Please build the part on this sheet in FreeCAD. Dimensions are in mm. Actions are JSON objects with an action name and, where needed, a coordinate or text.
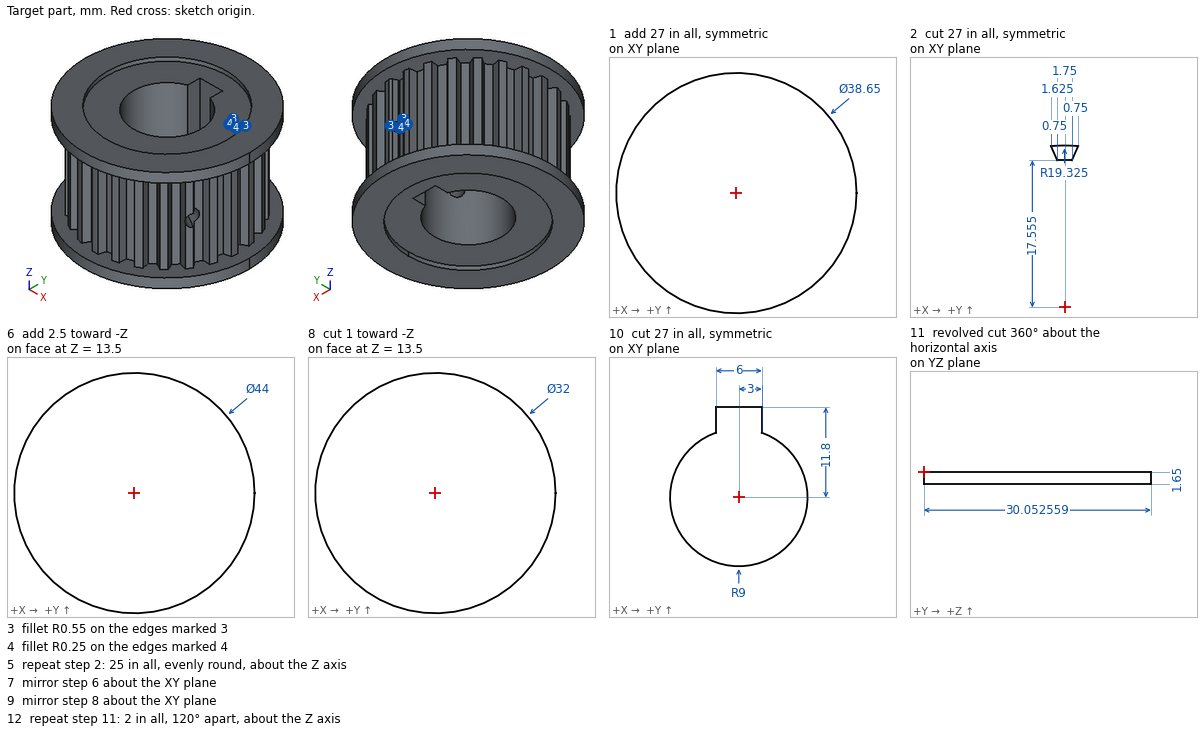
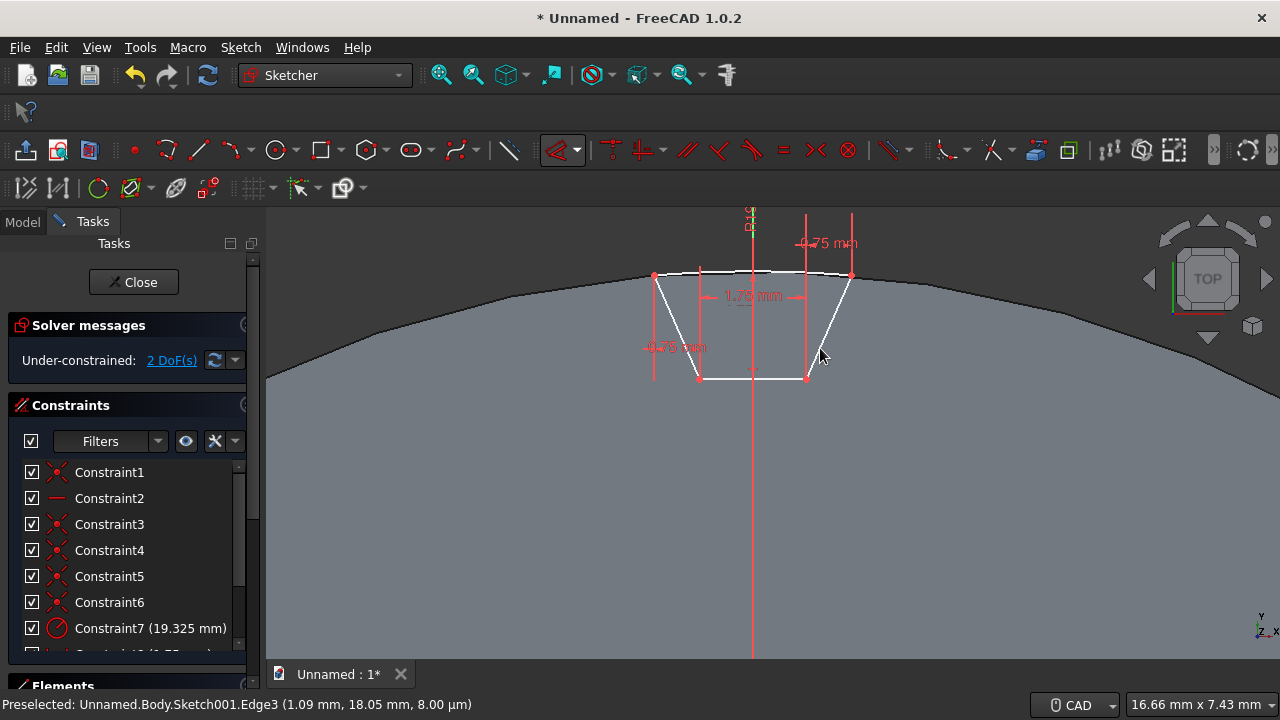
{"action": "left_click", "coordinate": [654, 276]}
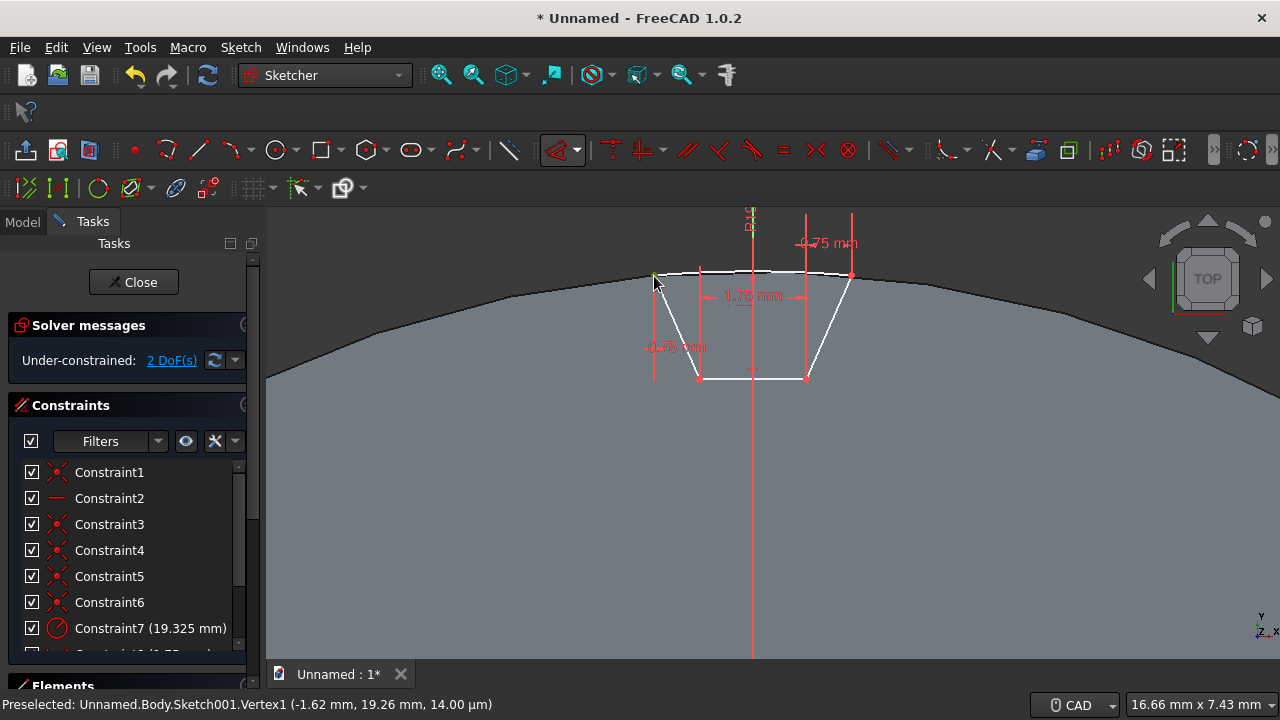
{"action": "left_click", "coordinate": [580, 150]}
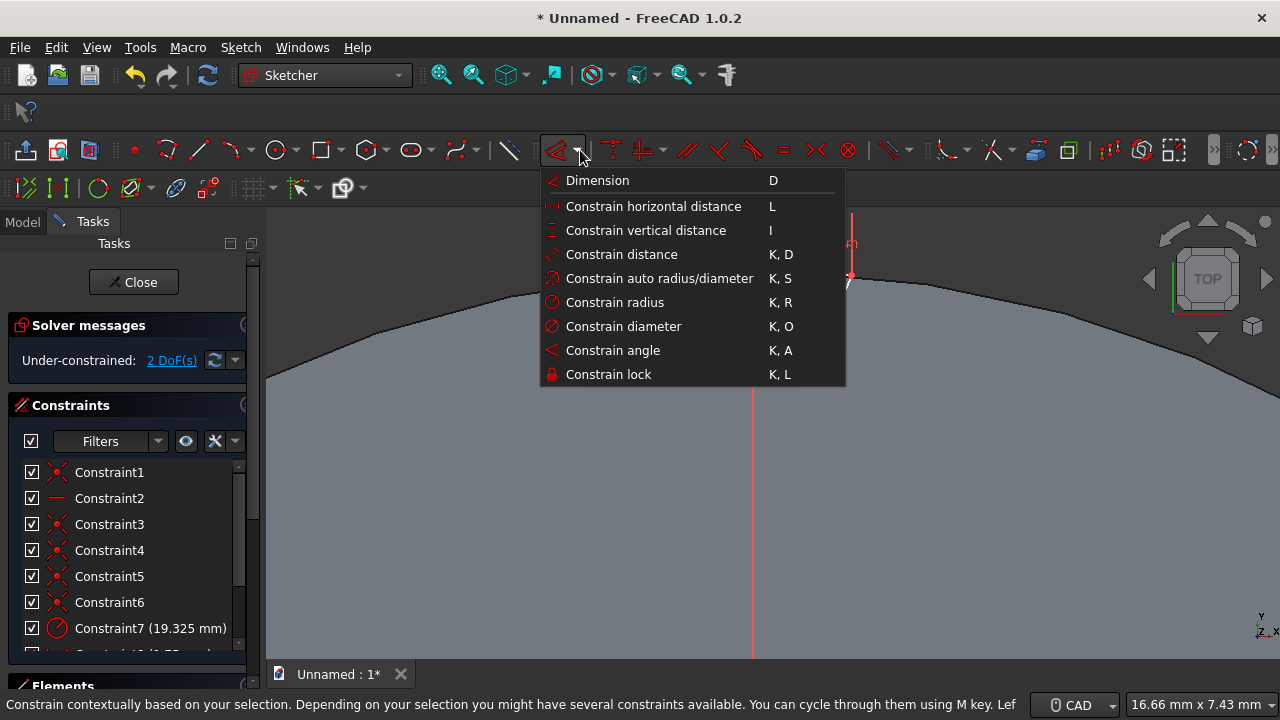
{"action": "left_click", "coordinate": [693, 206]}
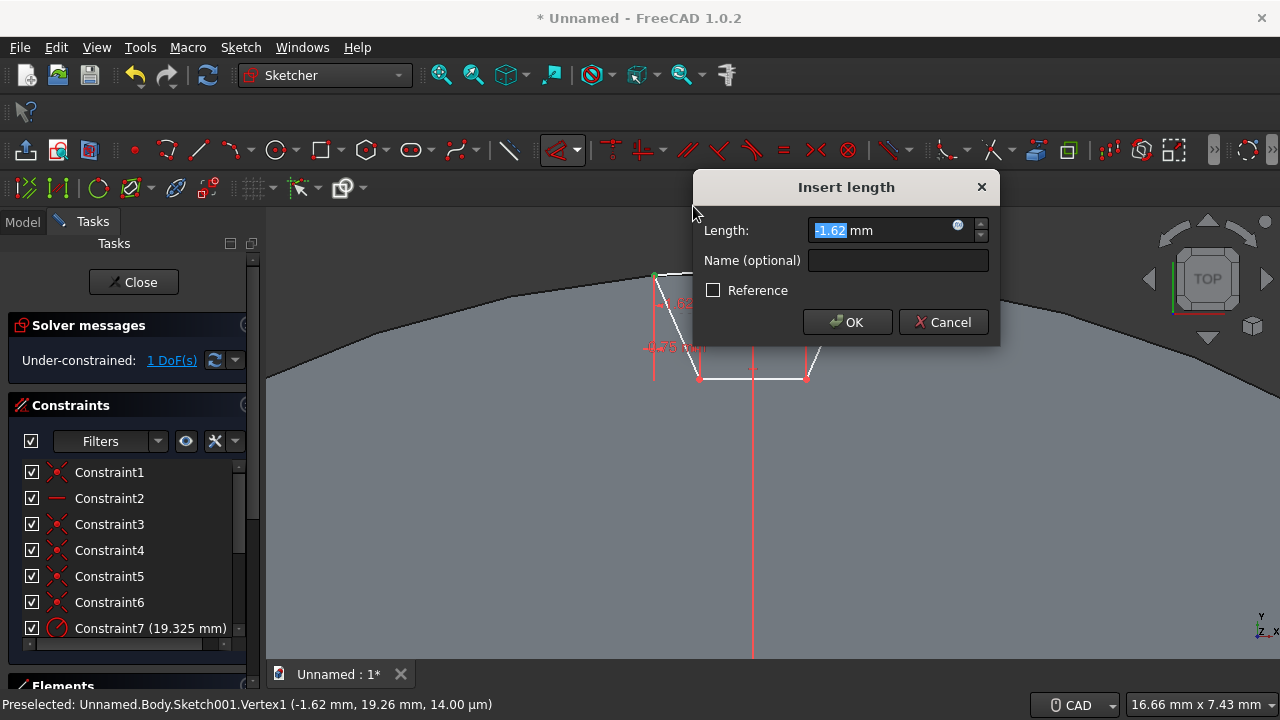
{"action": "type", "text": "-1.625"}
{"action": "key", "text": "Return"}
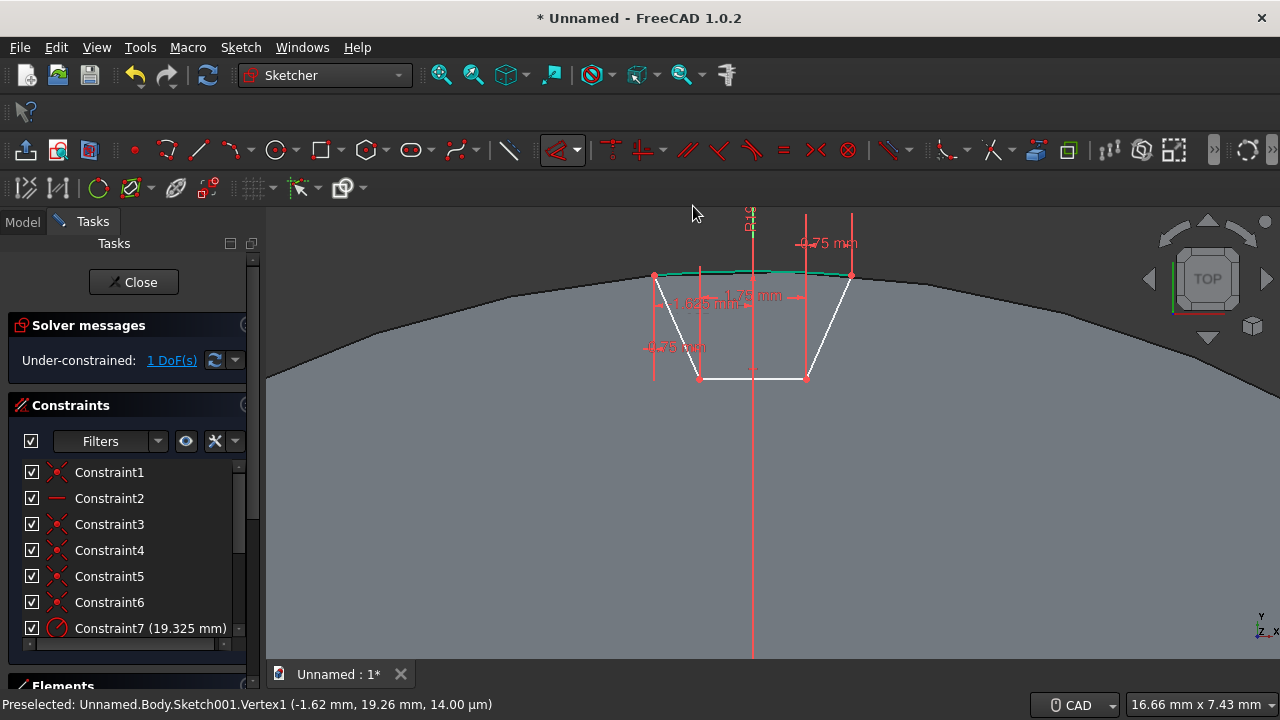
{"action": "left_click", "coordinate": [700, 379]}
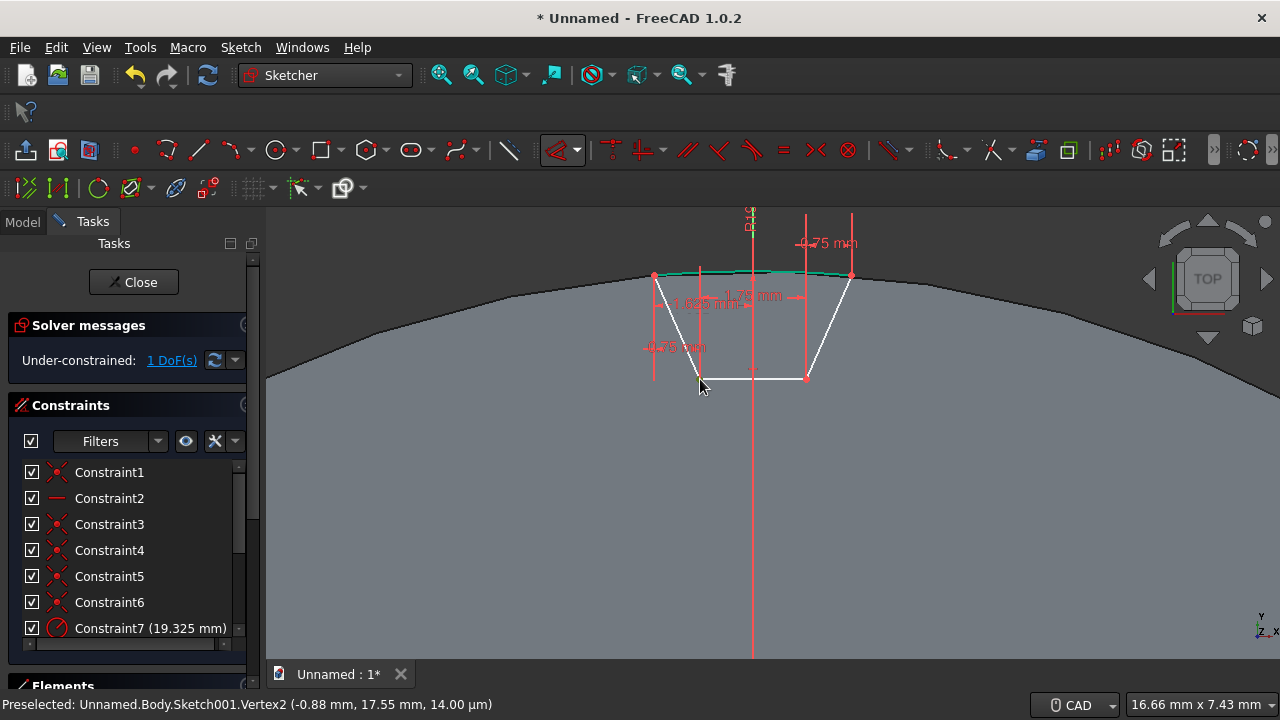
{"action": "left_click", "coordinate": [580, 150]}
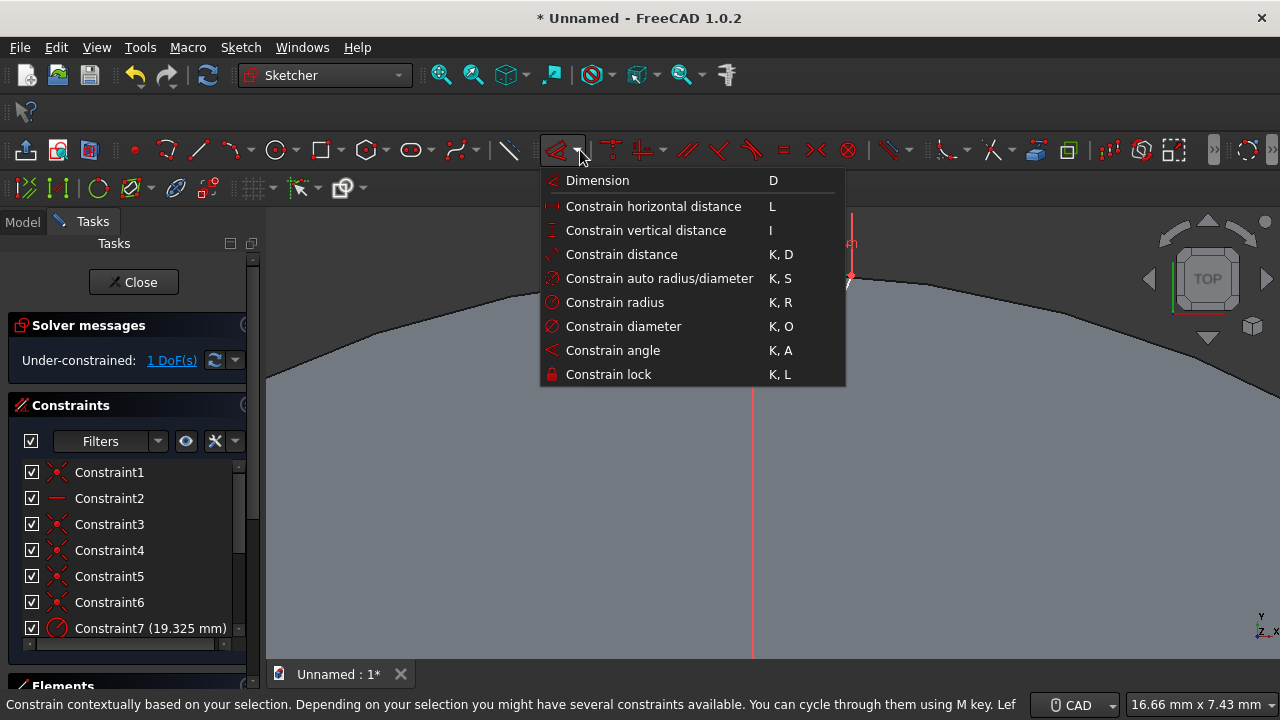
{"action": "left_click", "coordinate": [693, 230]}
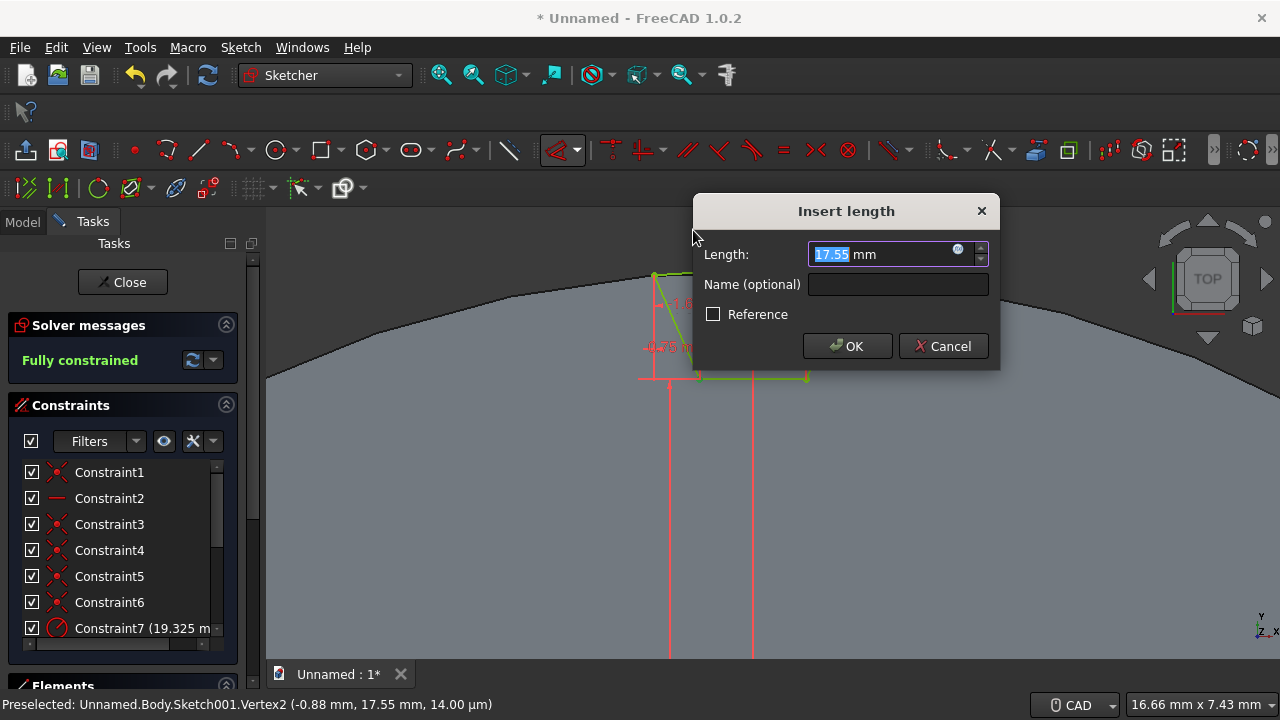
{"action": "type", "text": "17.555"}
{"action": "key", "text": "Return"}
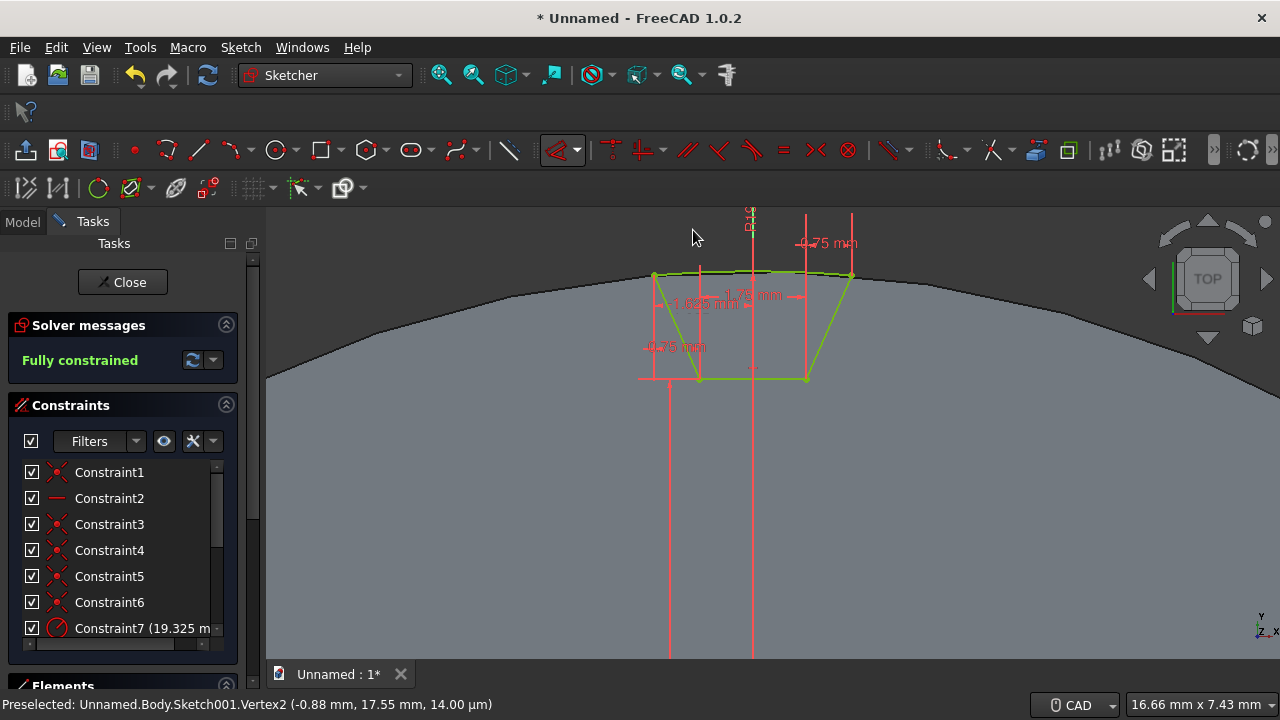
{"action": "left_click", "coordinate": [123, 282]}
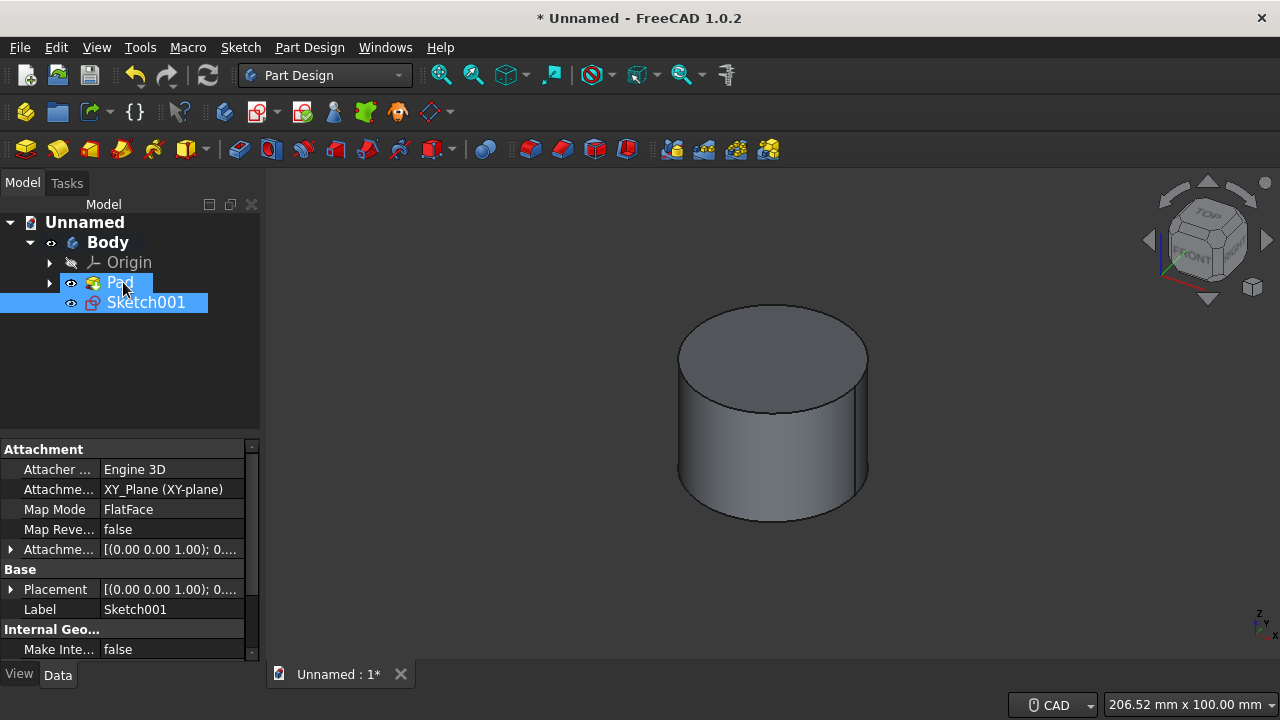
{"action": "left_click", "coordinate": [240, 150]}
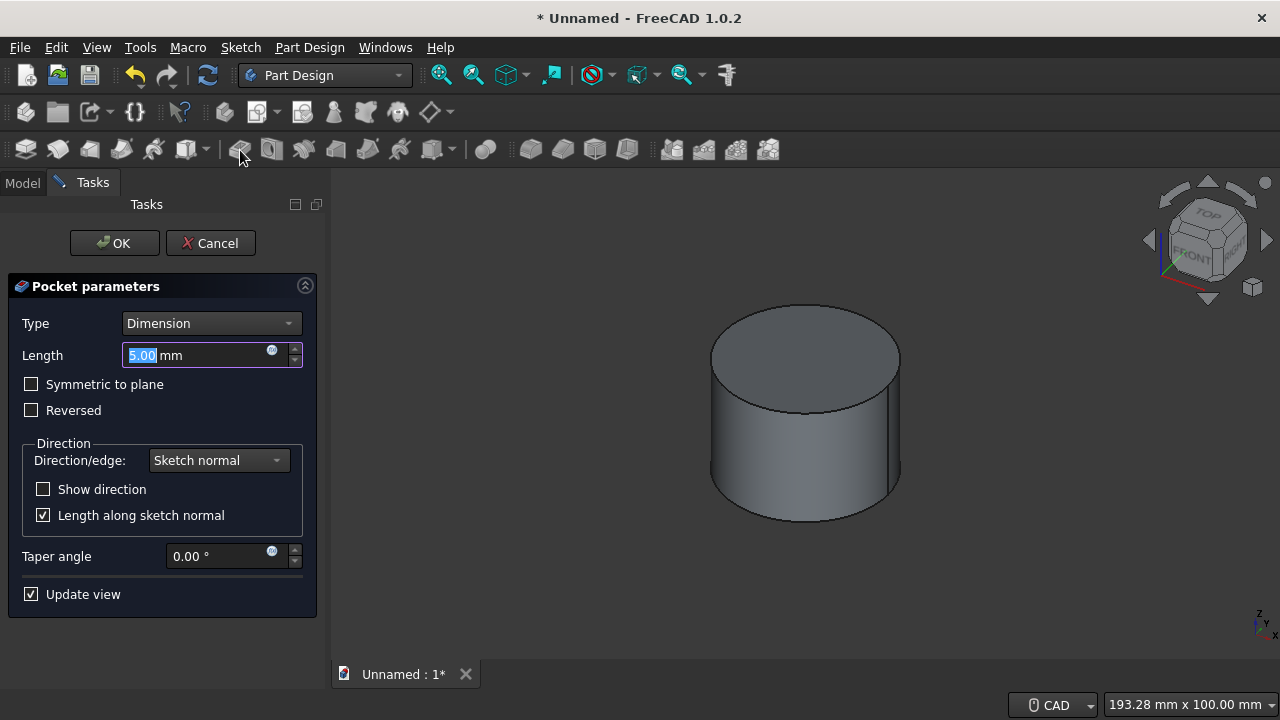
{"action": "type", "text": "27"}
{"action": "key", "text": "Tab"}